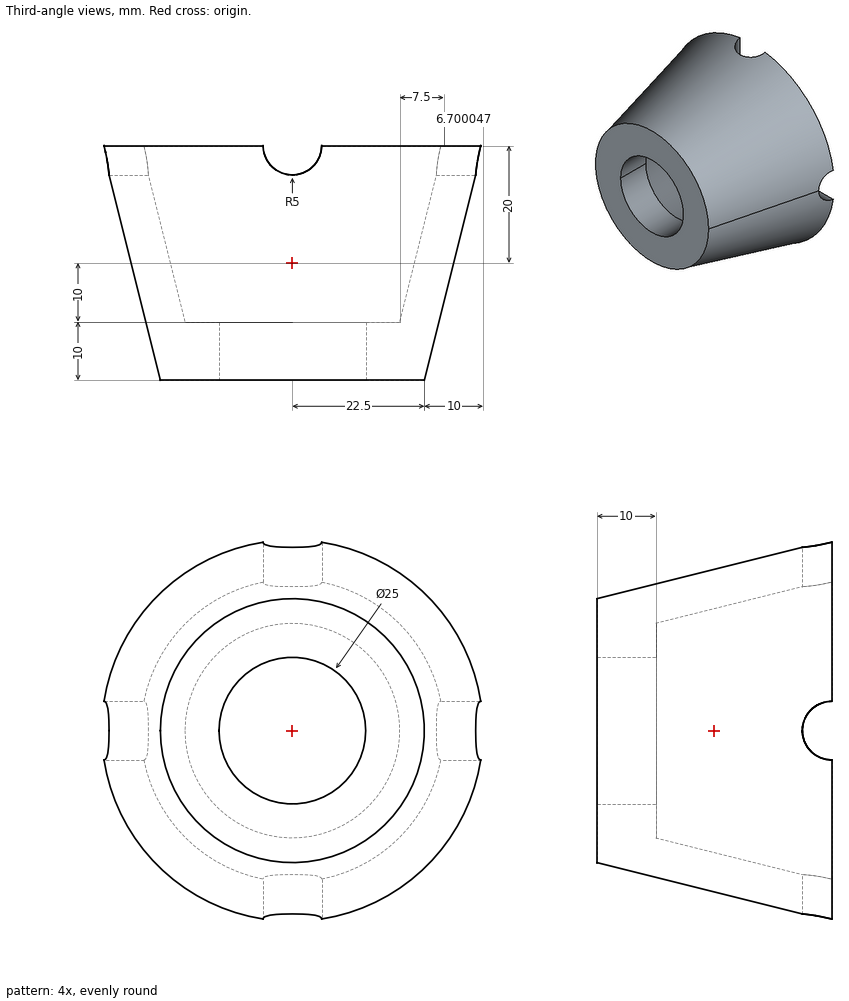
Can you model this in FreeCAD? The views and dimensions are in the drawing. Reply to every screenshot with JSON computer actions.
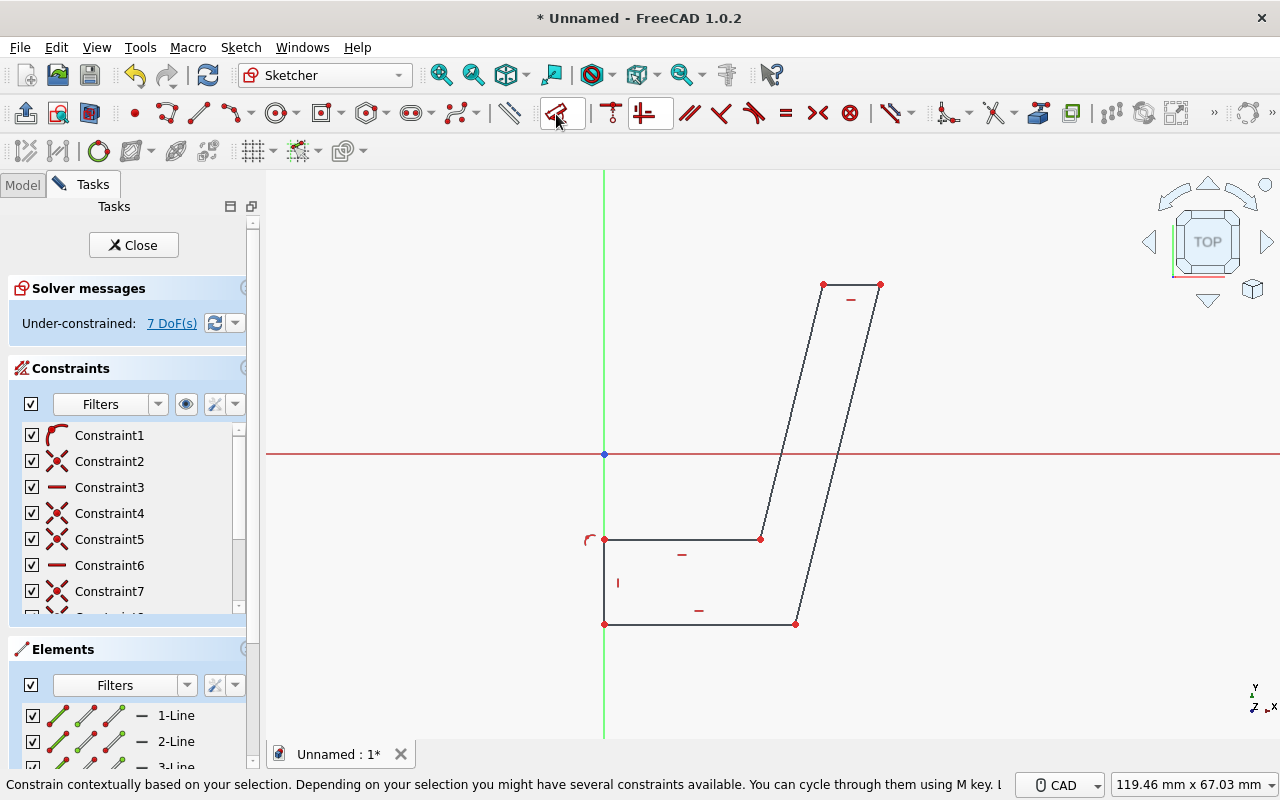
{"action": "left_click", "coordinate": [604, 565]}
{"action": "left_click", "coordinate": [570, 582]}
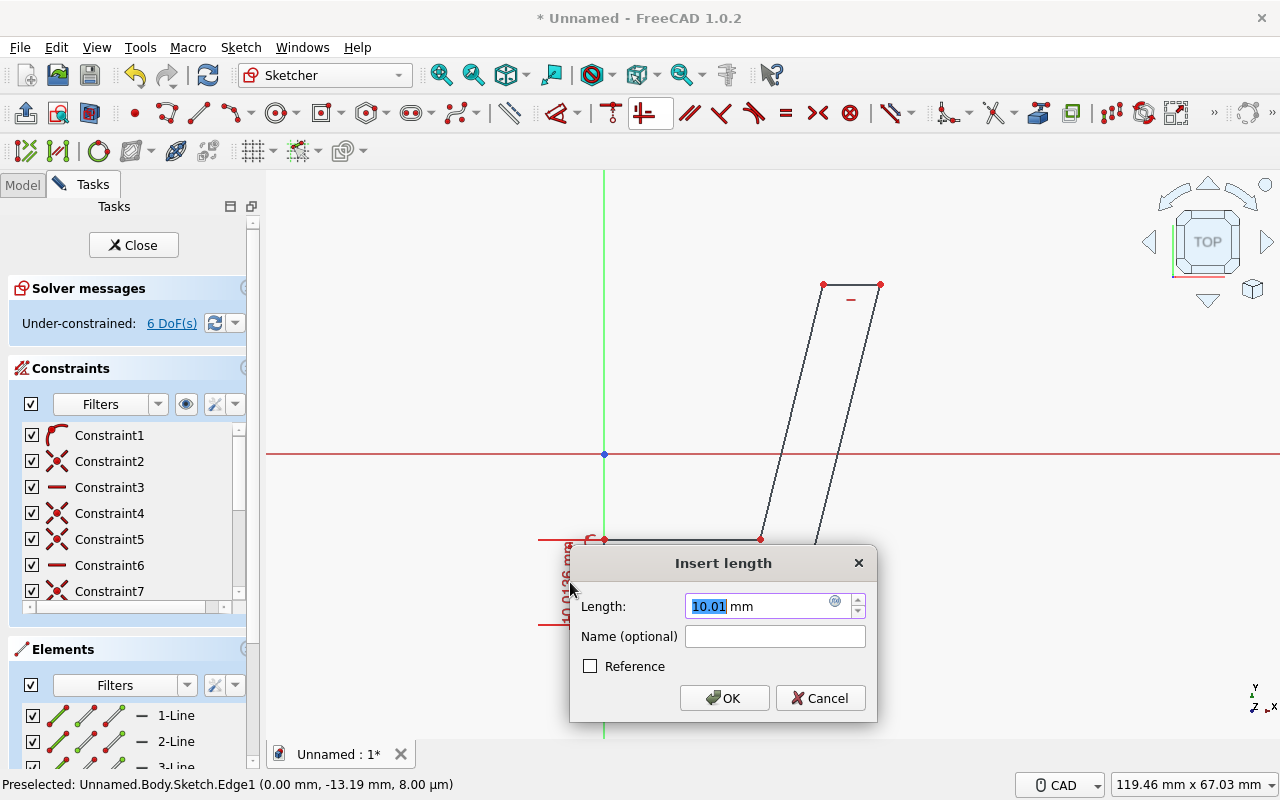
{"action": "type", "text": "10"}
{"action": "key", "text": "Return"}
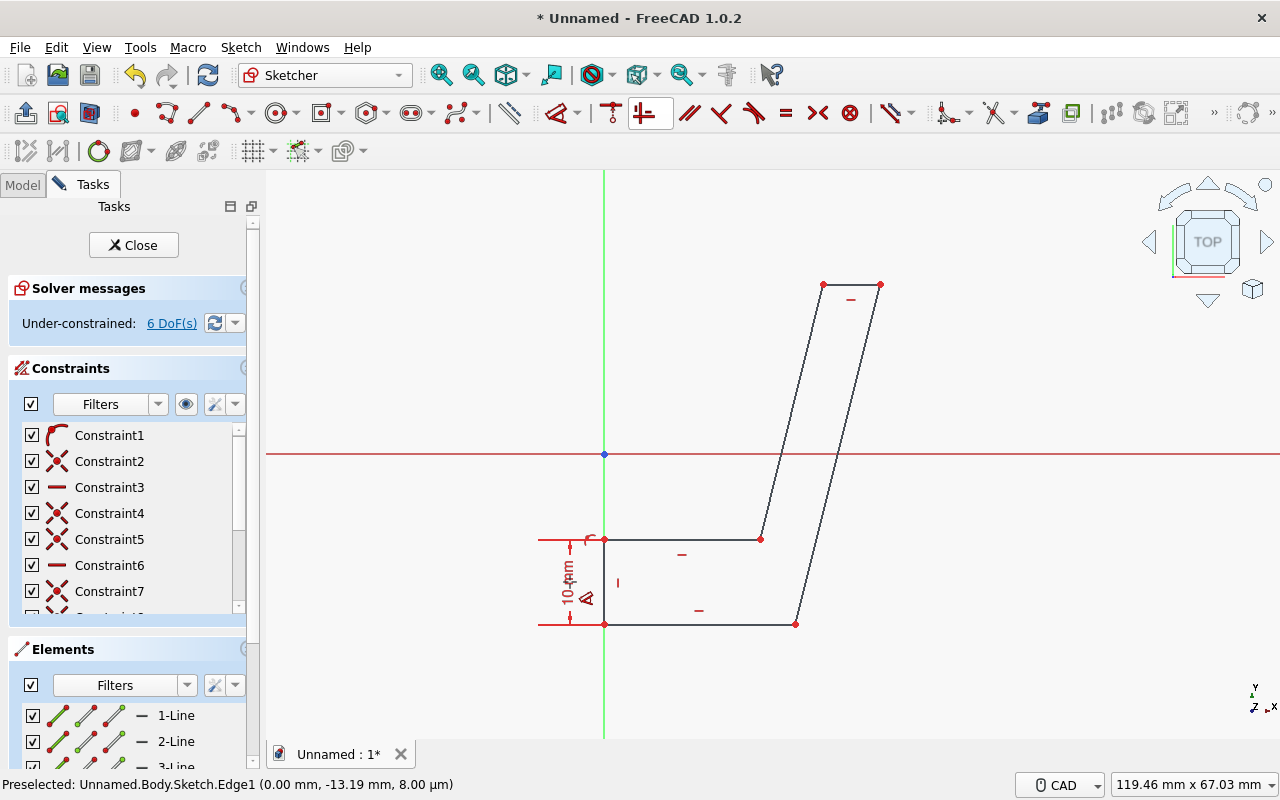
{"action": "left_click", "coordinate": [604, 540]}
{"action": "left_click", "coordinate": [570, 497]}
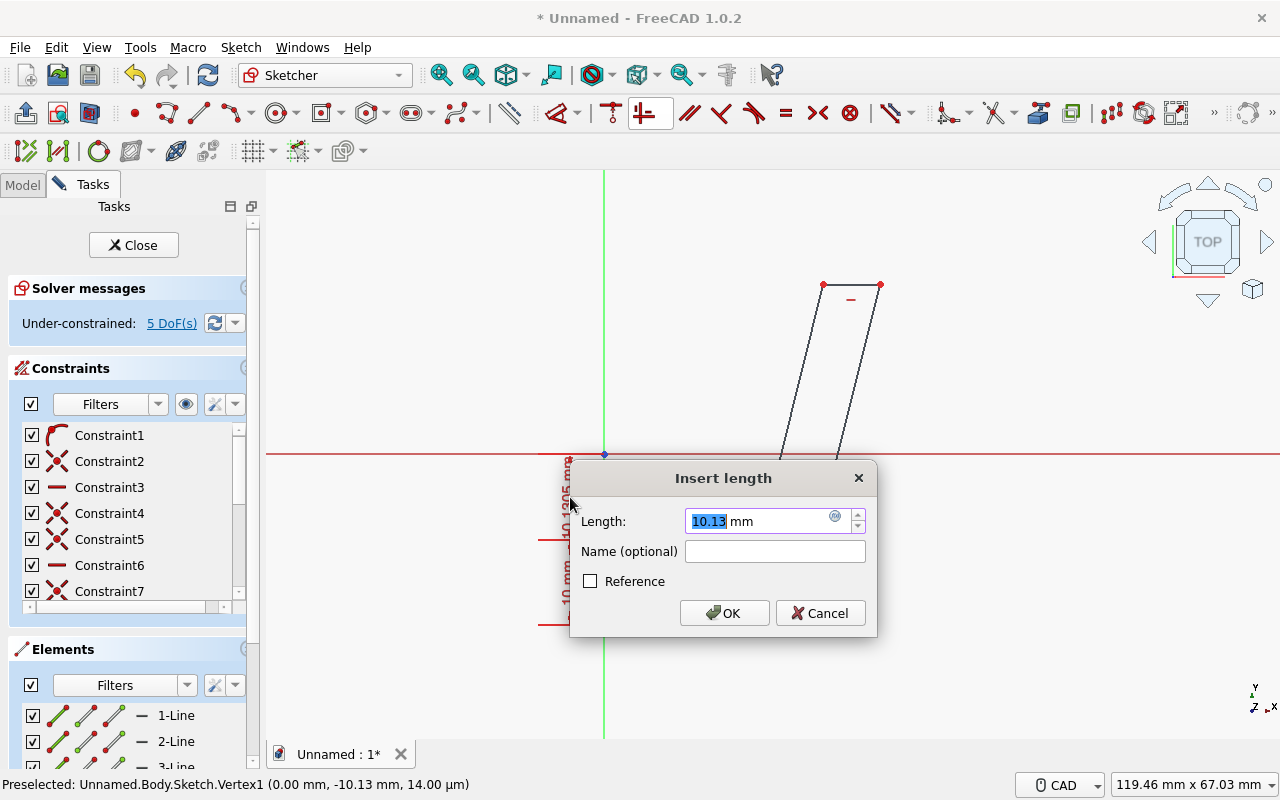
{"action": "type", "text": "10"}
{"action": "key", "text": "Return"}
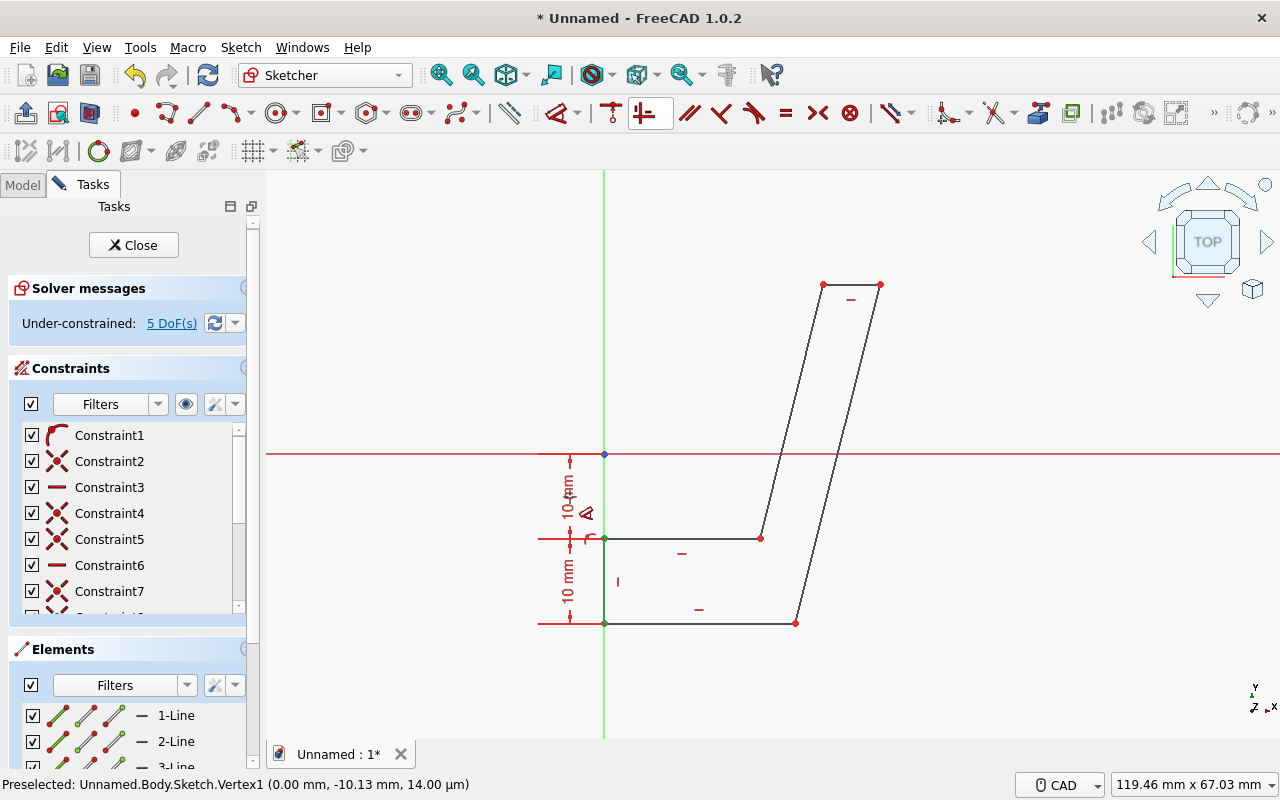
{"action": "left_click", "coordinate": [880, 285]}
{"action": "left_click", "coordinate": [570, 370]}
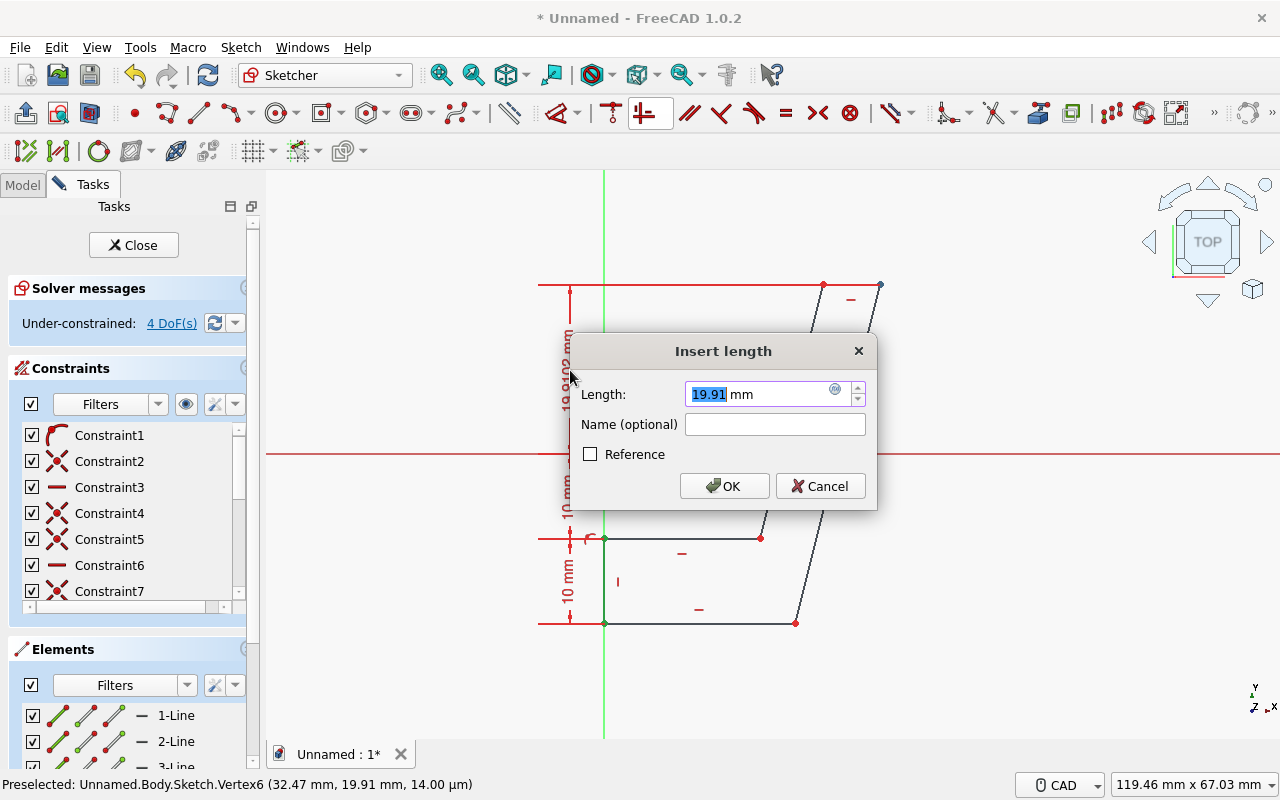
{"action": "type", "text": "20"}
{"action": "key", "text": "Return"}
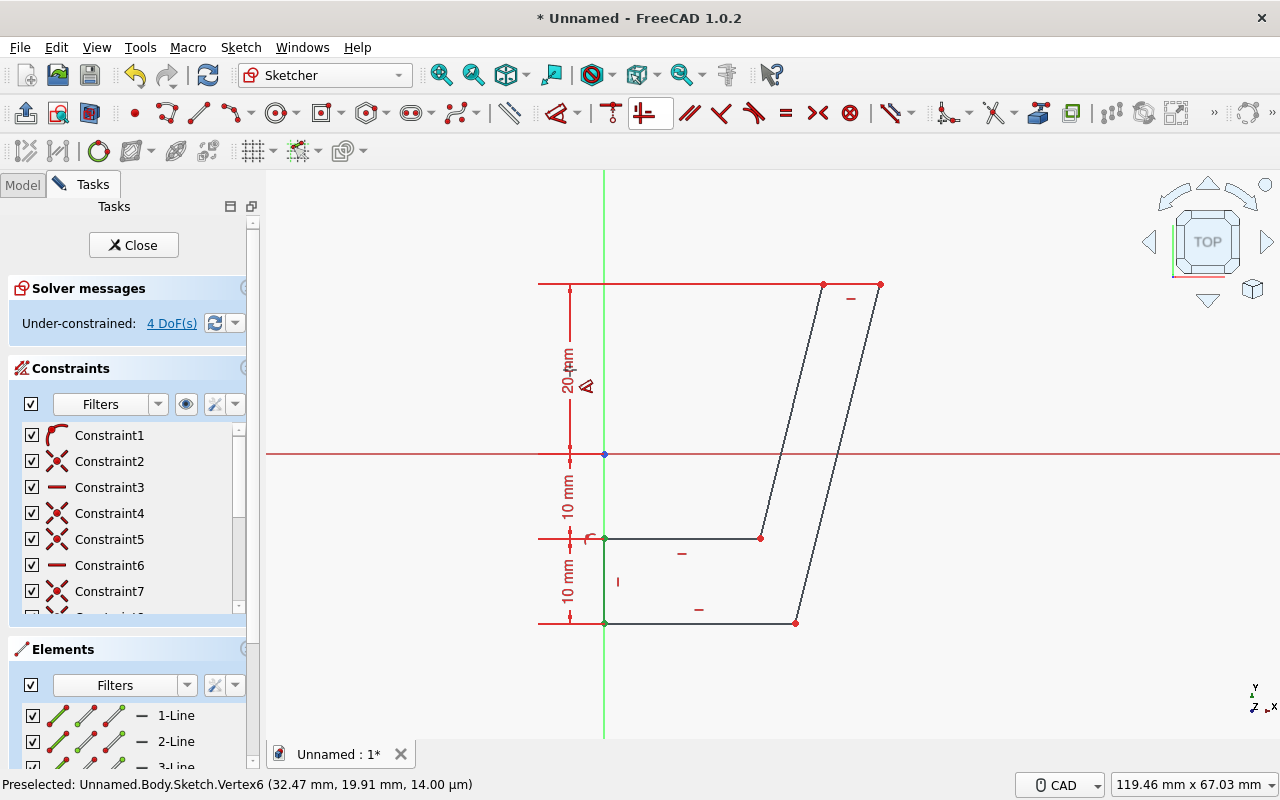
{"action": "left_click", "coordinate": [821, 522]}
{"action": "left_click", "coordinate": [838, 658]}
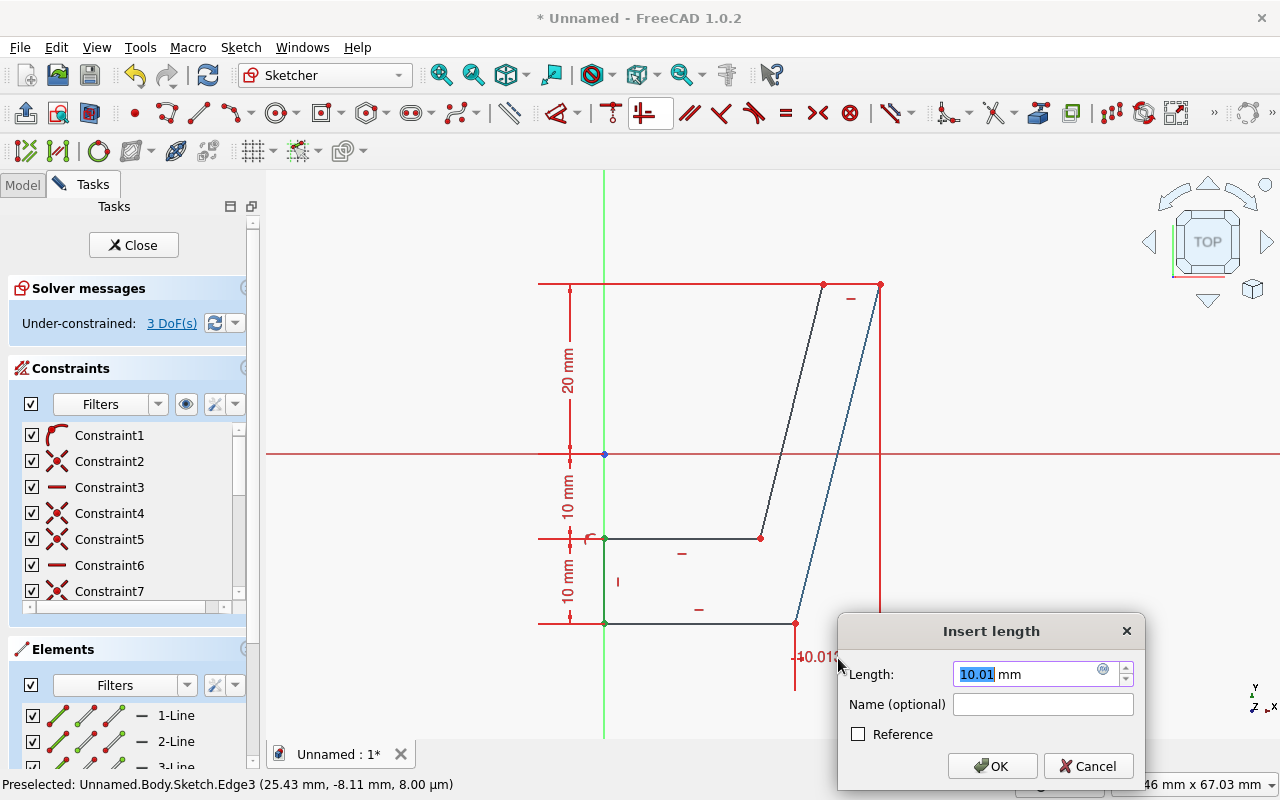
{"action": "type", "text": "10"}
{"action": "key", "text": "Return"}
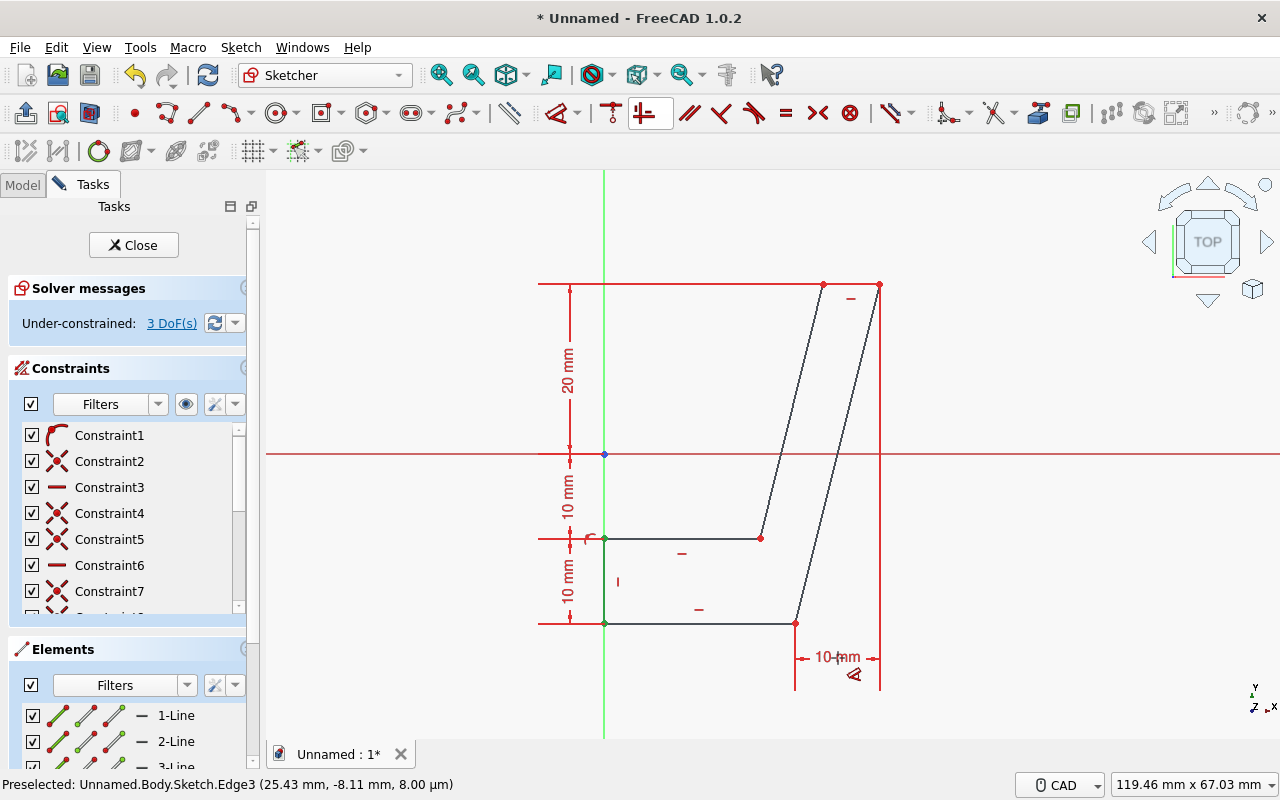
{"action": "left_click", "coordinate": [662, 624]}
{"action": "left_click", "coordinate": [700, 658]}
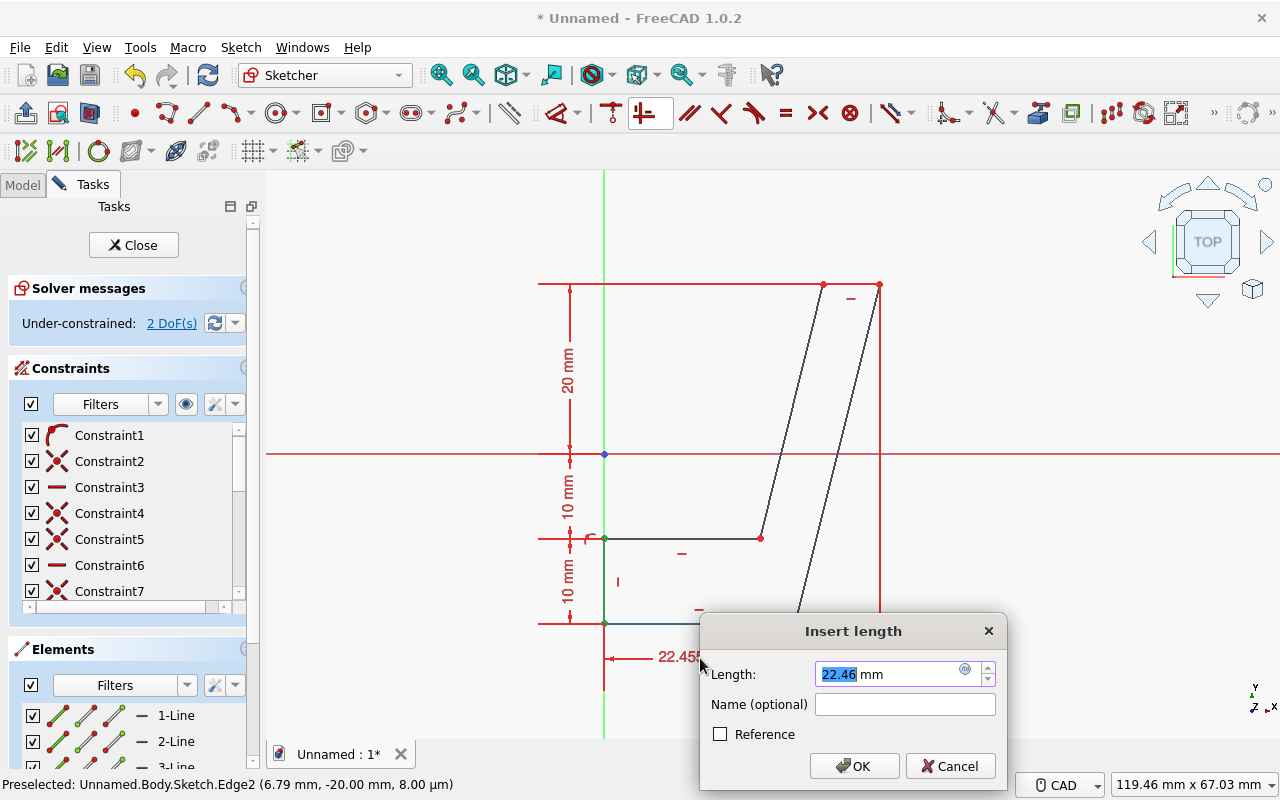
{"action": "type", "text": "22.5"}
{"action": "key", "text": "Return"}